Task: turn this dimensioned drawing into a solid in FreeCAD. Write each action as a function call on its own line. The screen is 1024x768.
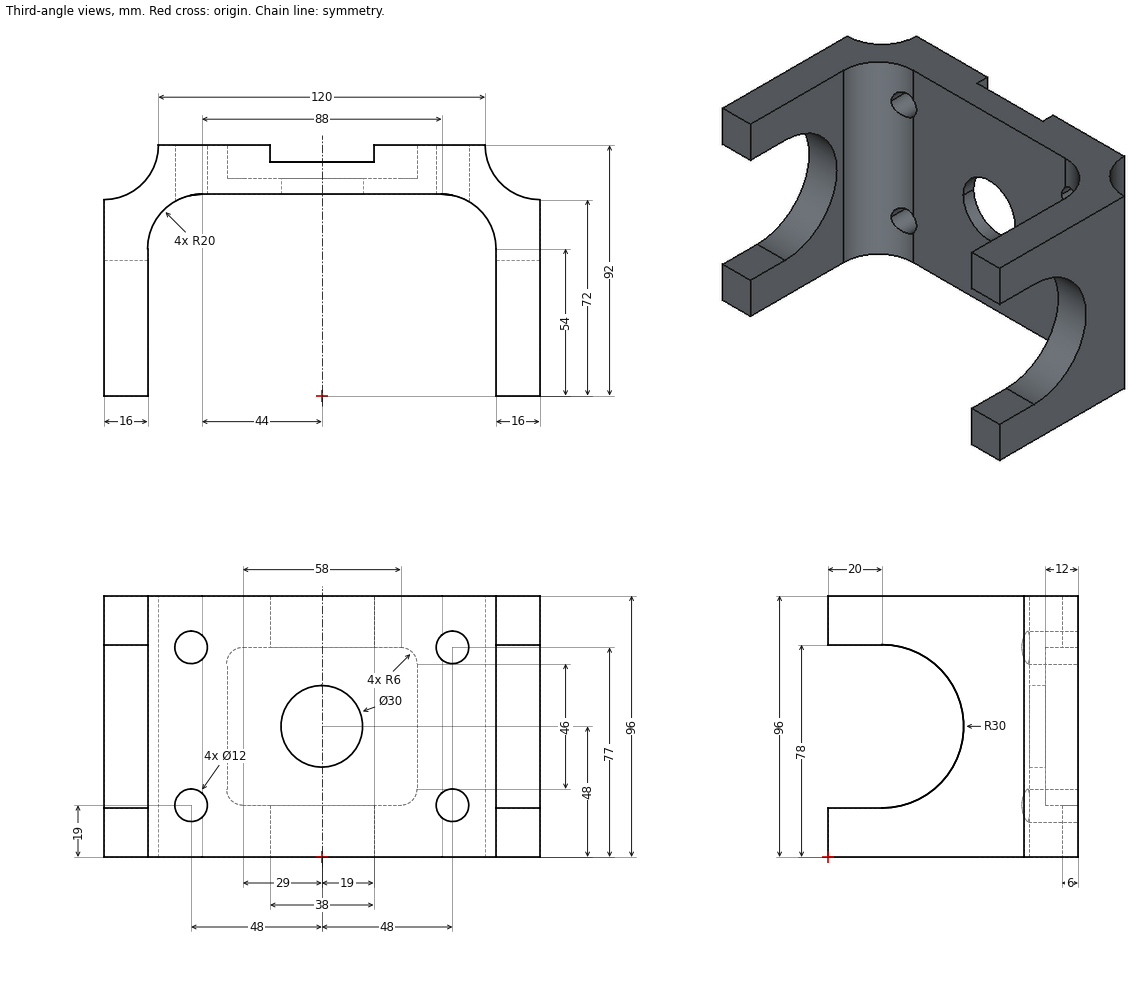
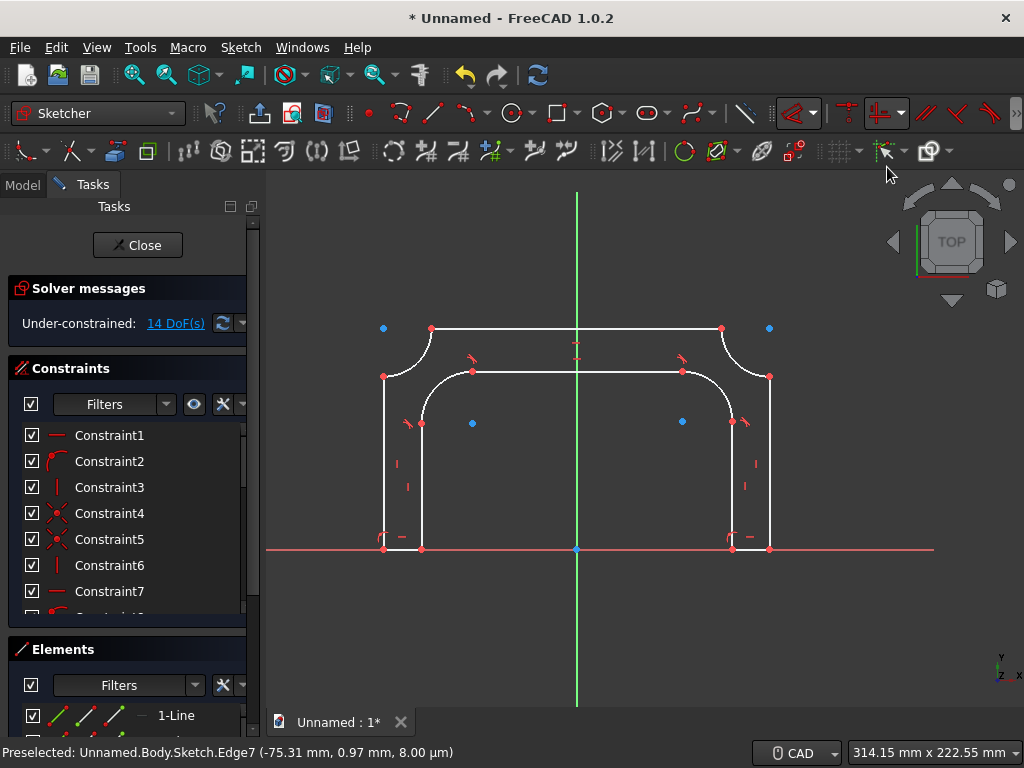
click(727, 399)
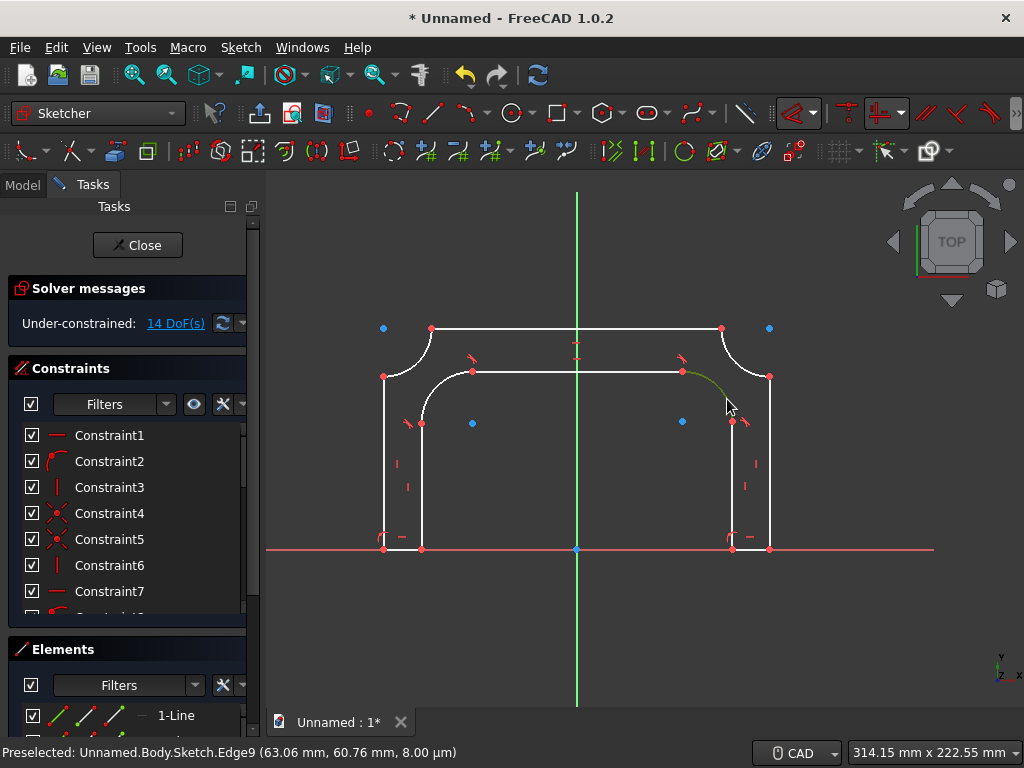
click(727, 350)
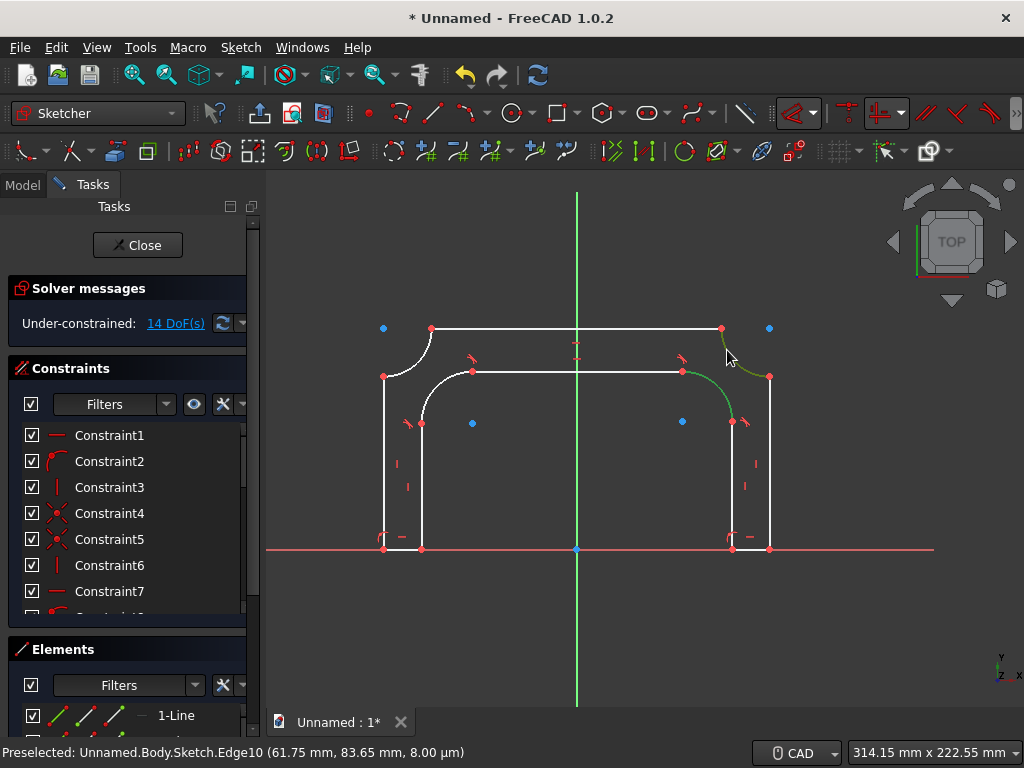
click(405, 371)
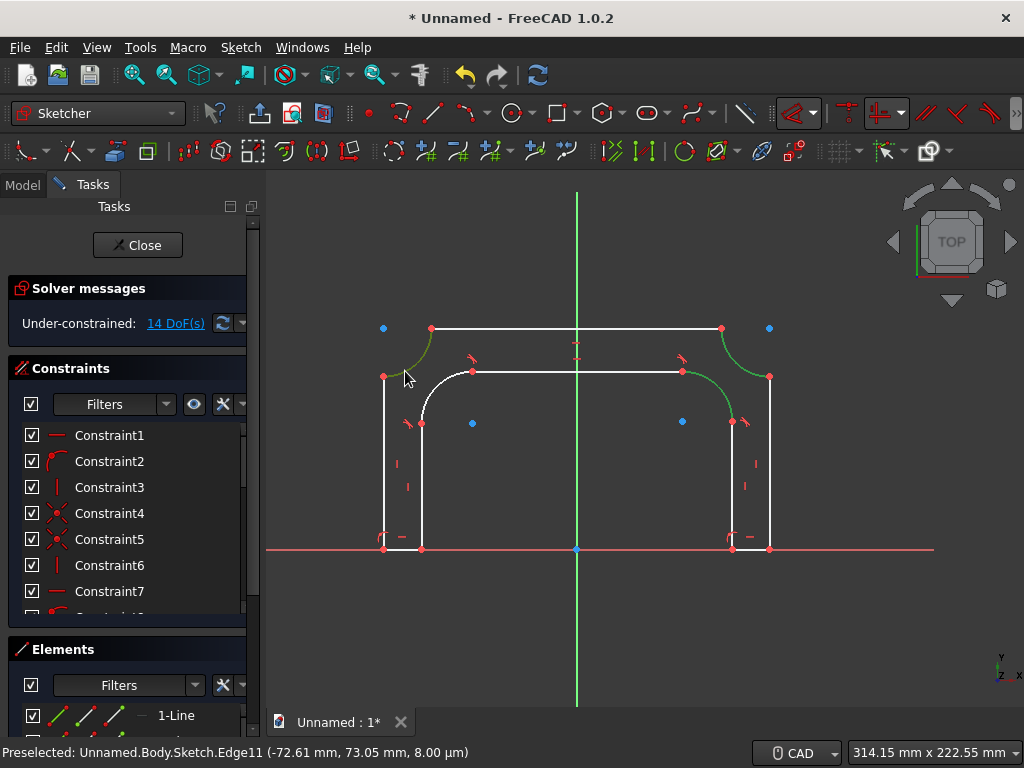
click(450, 377)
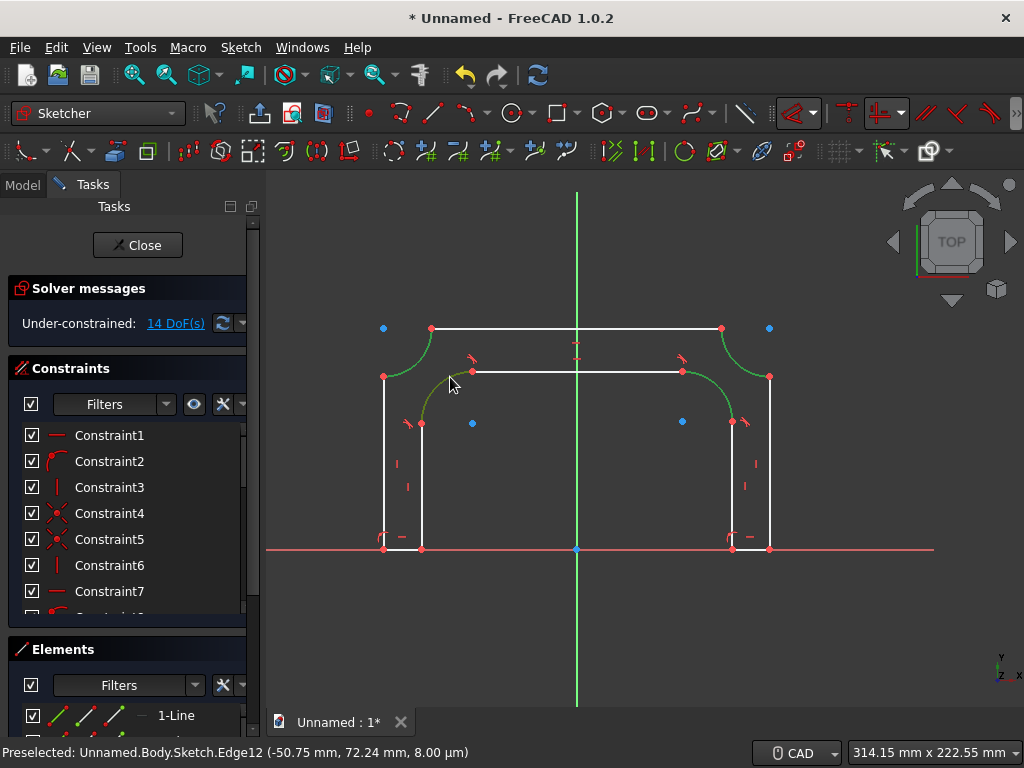
key(e)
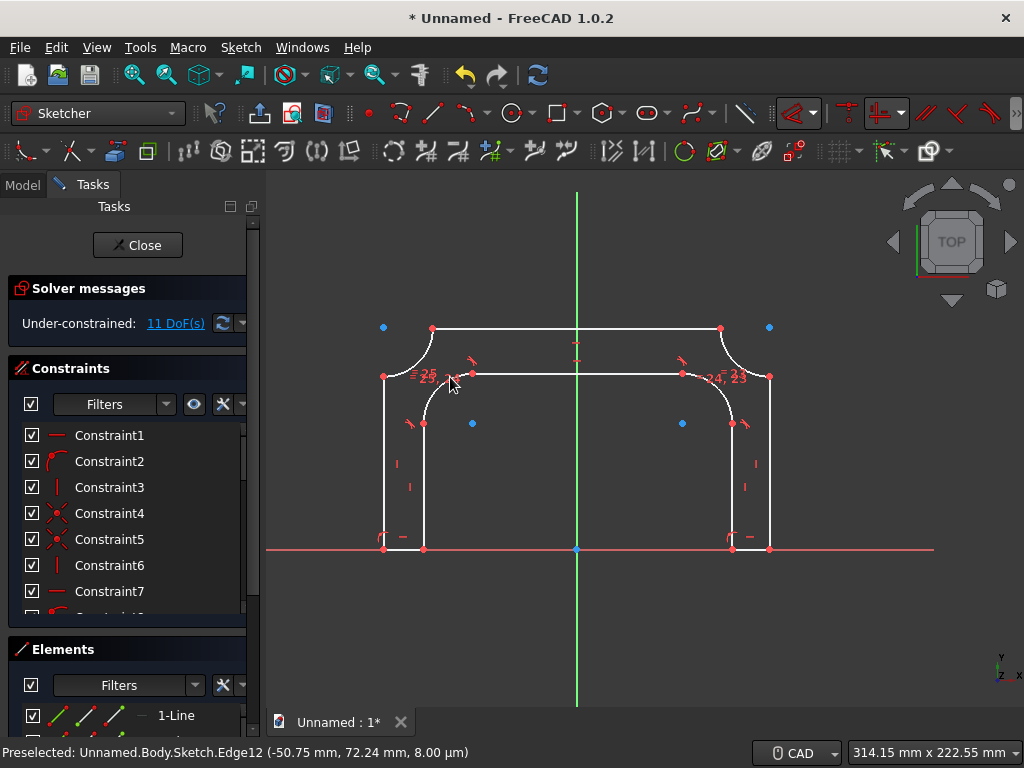
click(769, 328)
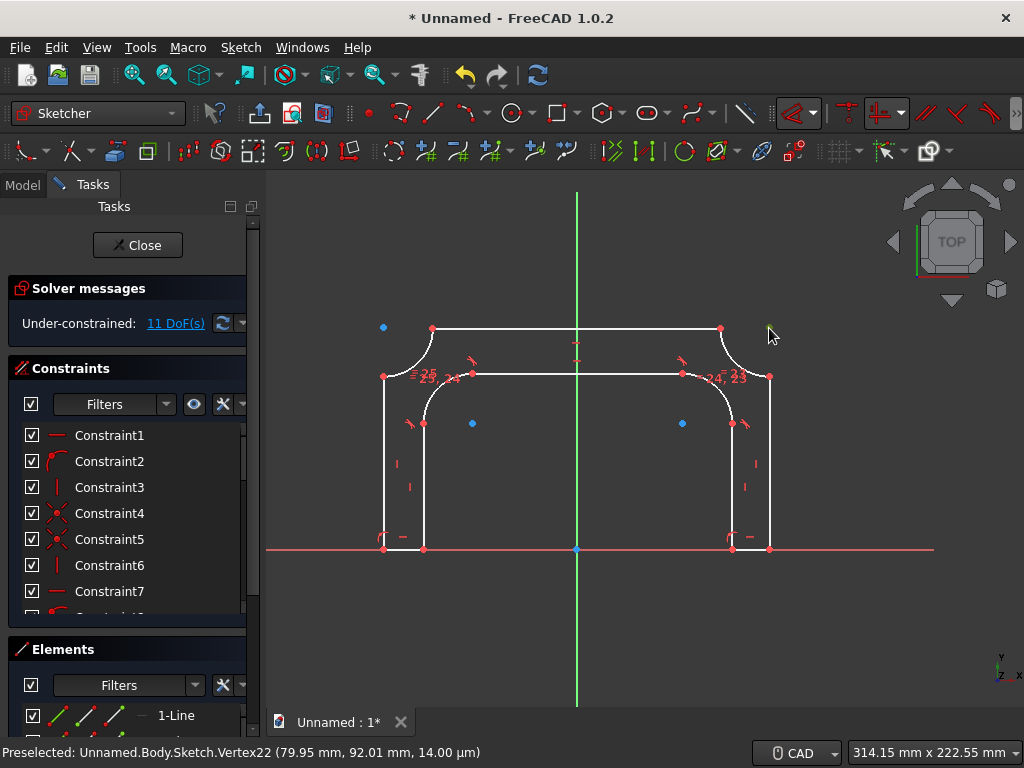
click(384, 328)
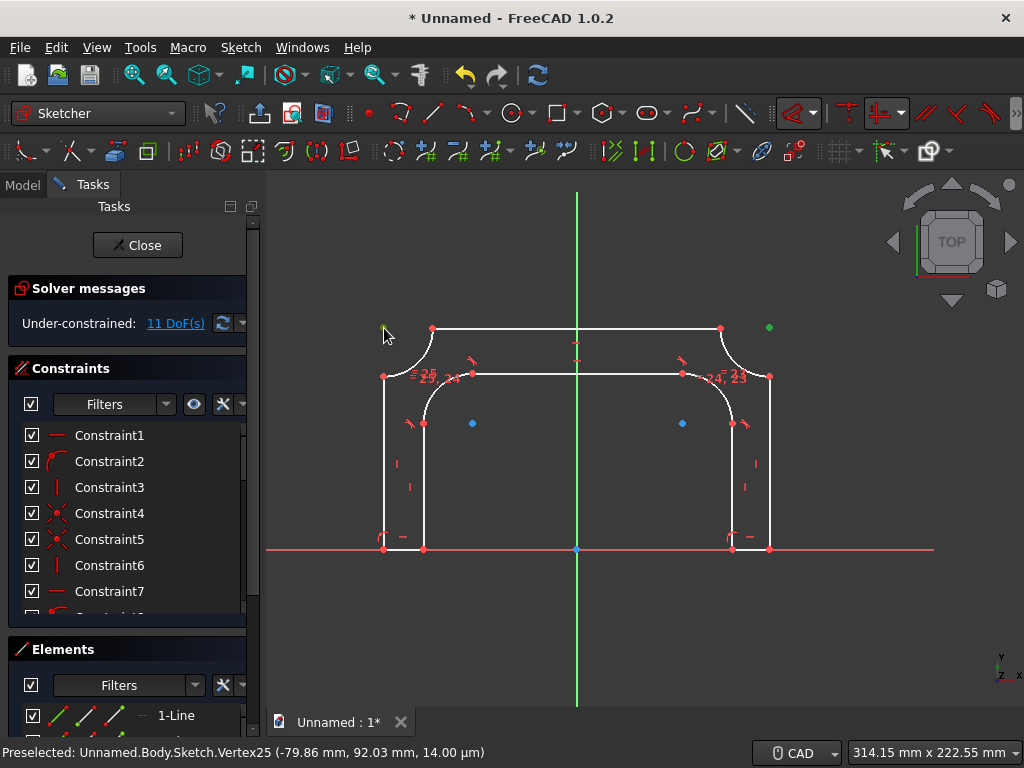
click(577, 645)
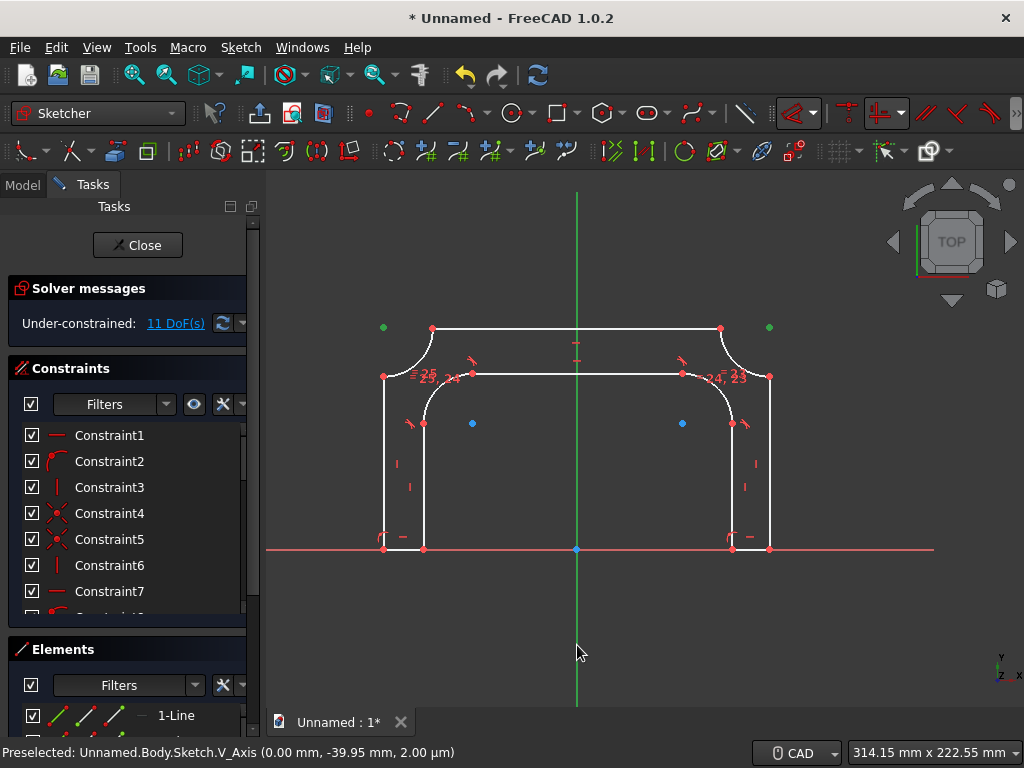
key(s)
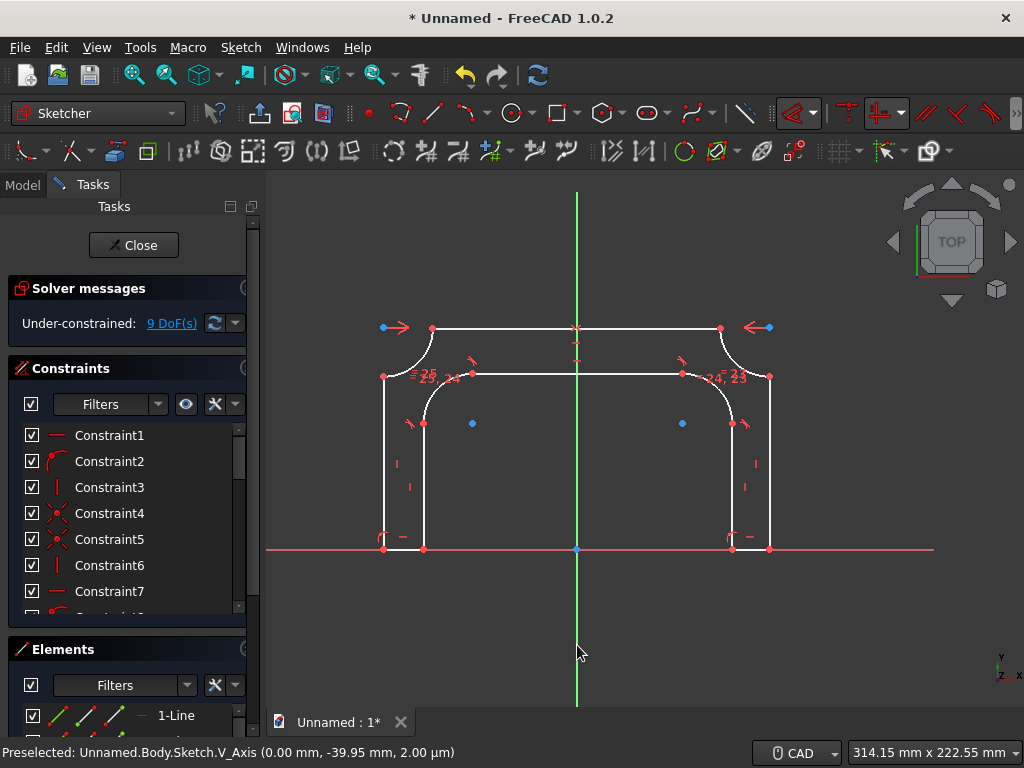
click(792, 114)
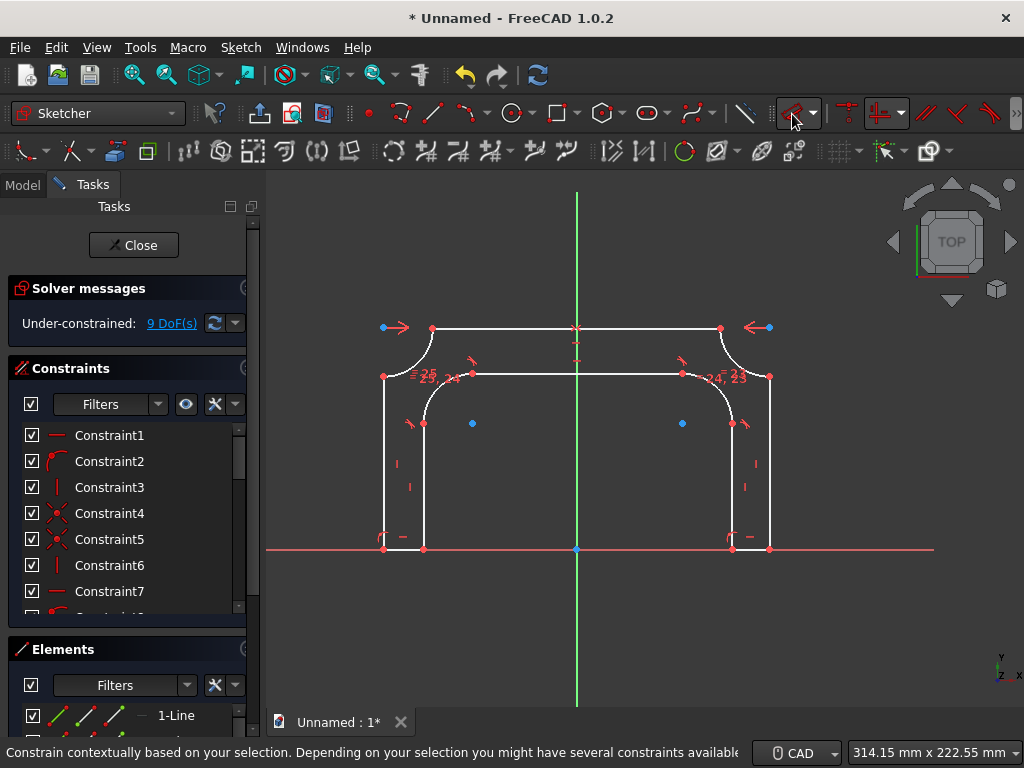
click(727, 401)
click(753, 465)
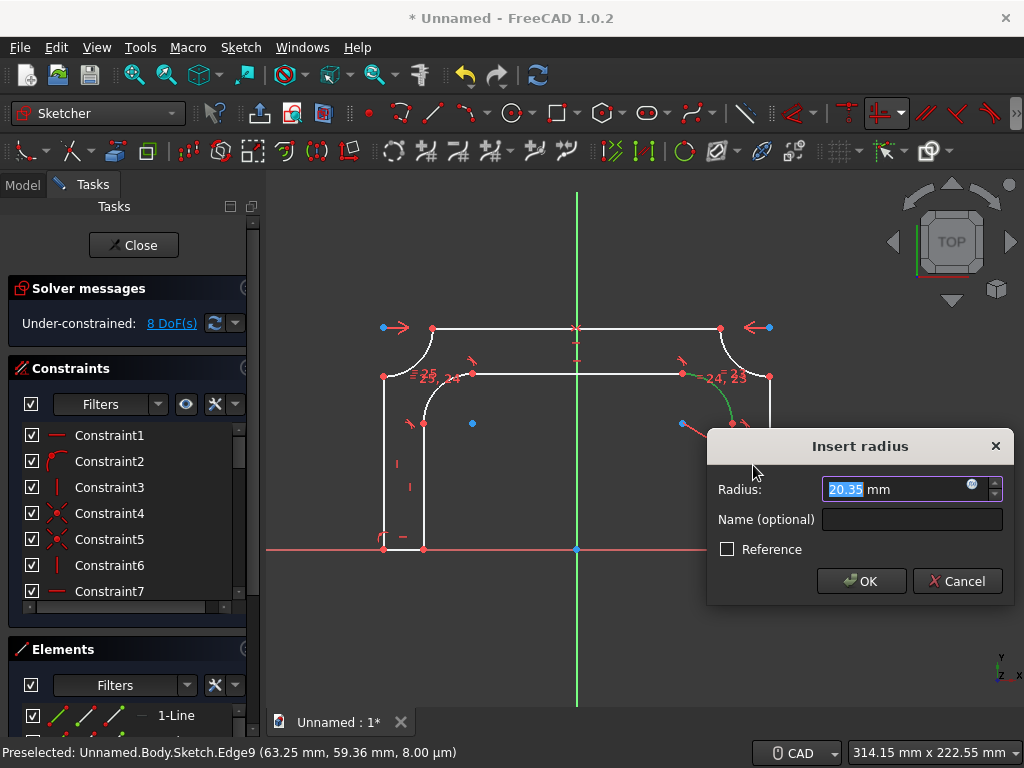
text(20)
key(Return)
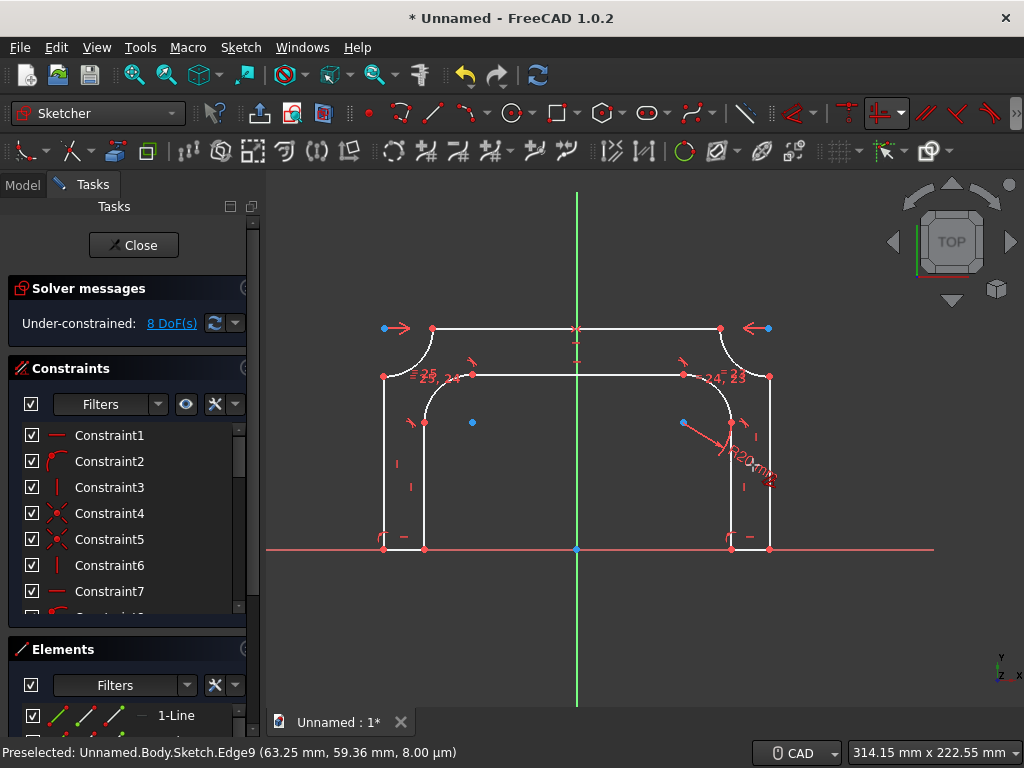
click(536, 375)
click(530, 409)